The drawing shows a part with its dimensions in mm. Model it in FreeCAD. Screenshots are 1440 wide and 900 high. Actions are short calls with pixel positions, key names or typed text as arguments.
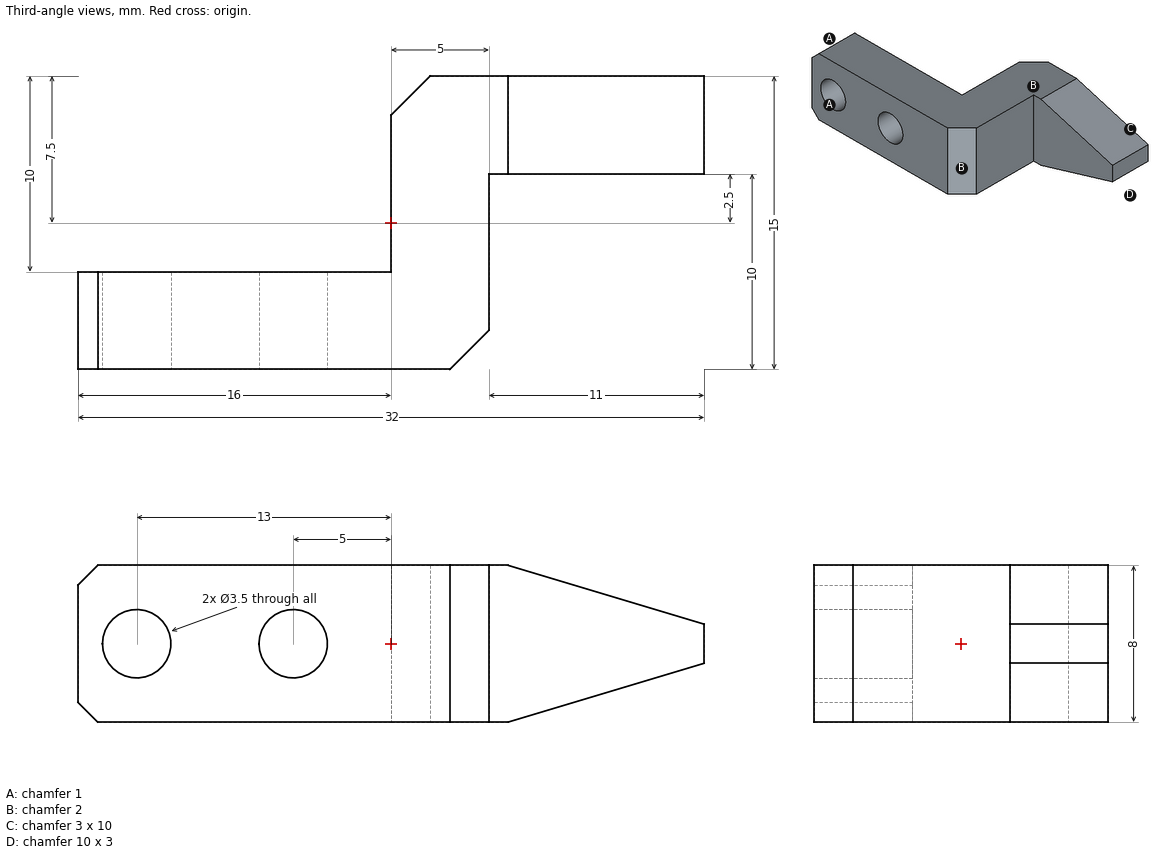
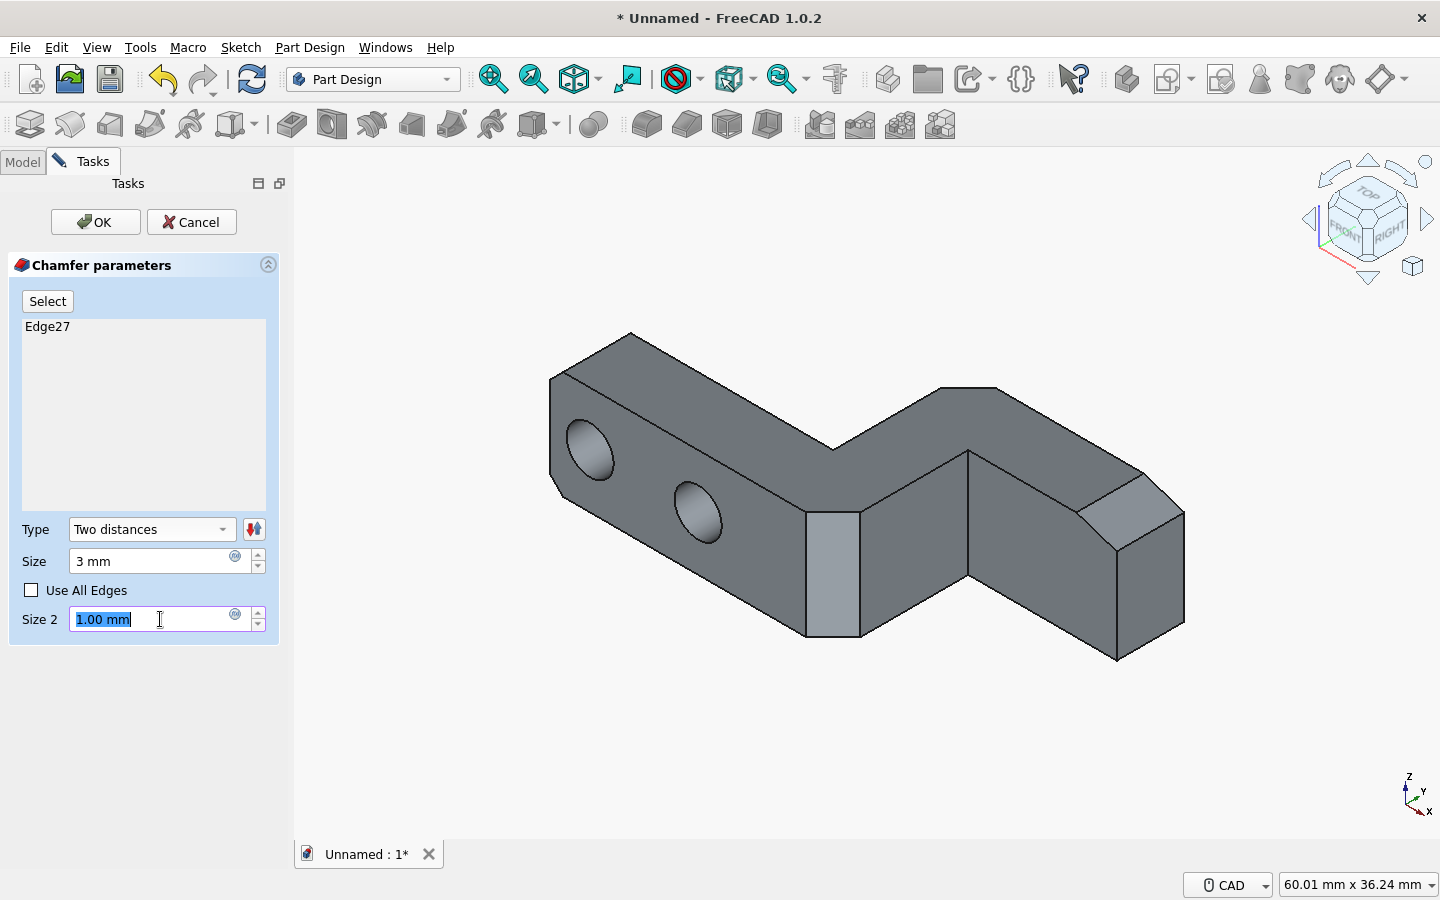
text(10)
key(Tab)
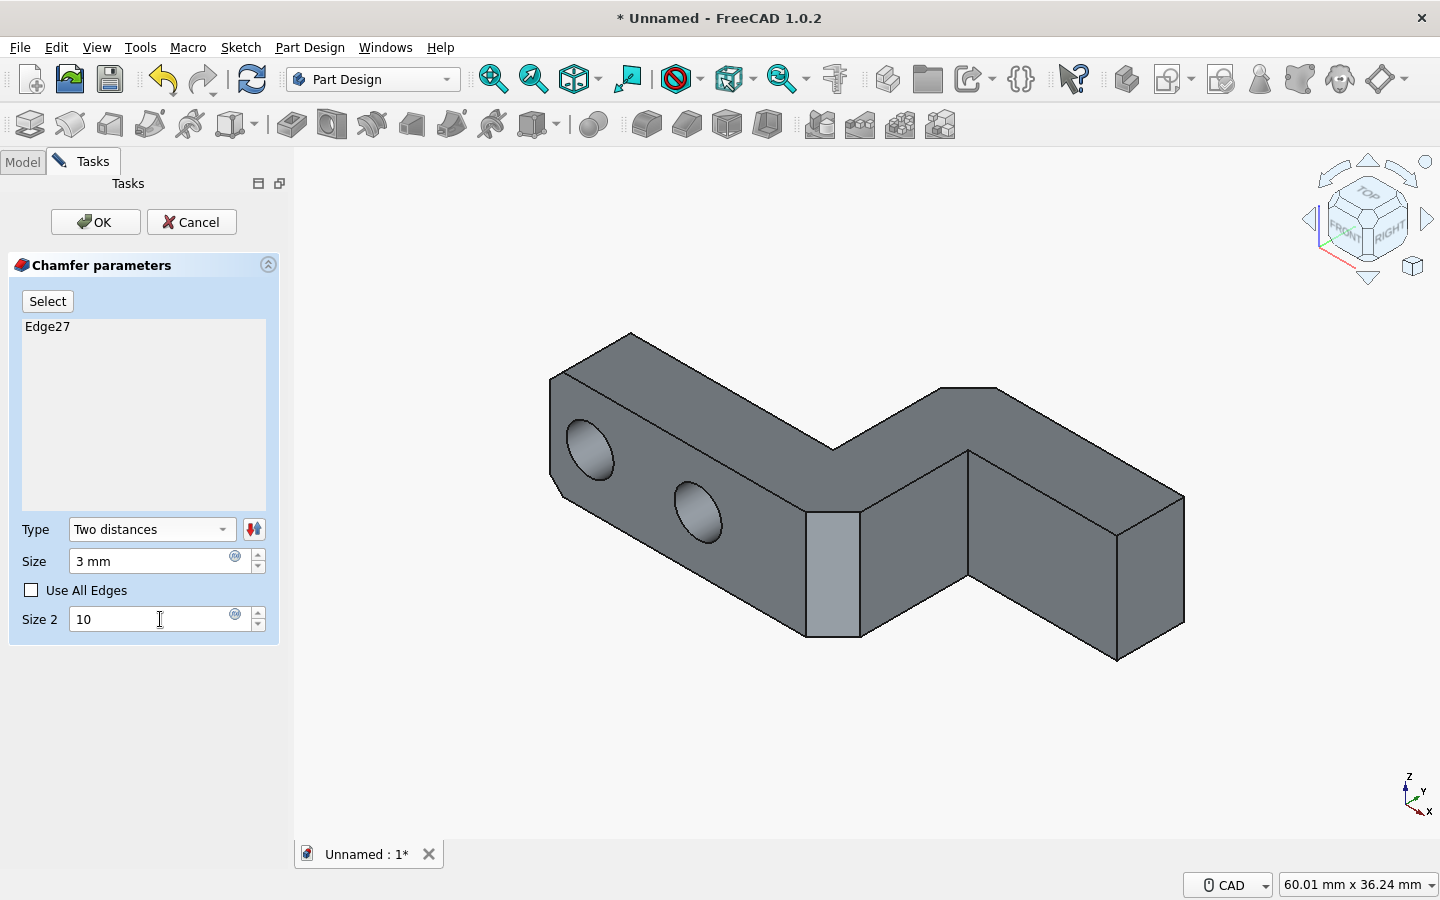
click(254, 530)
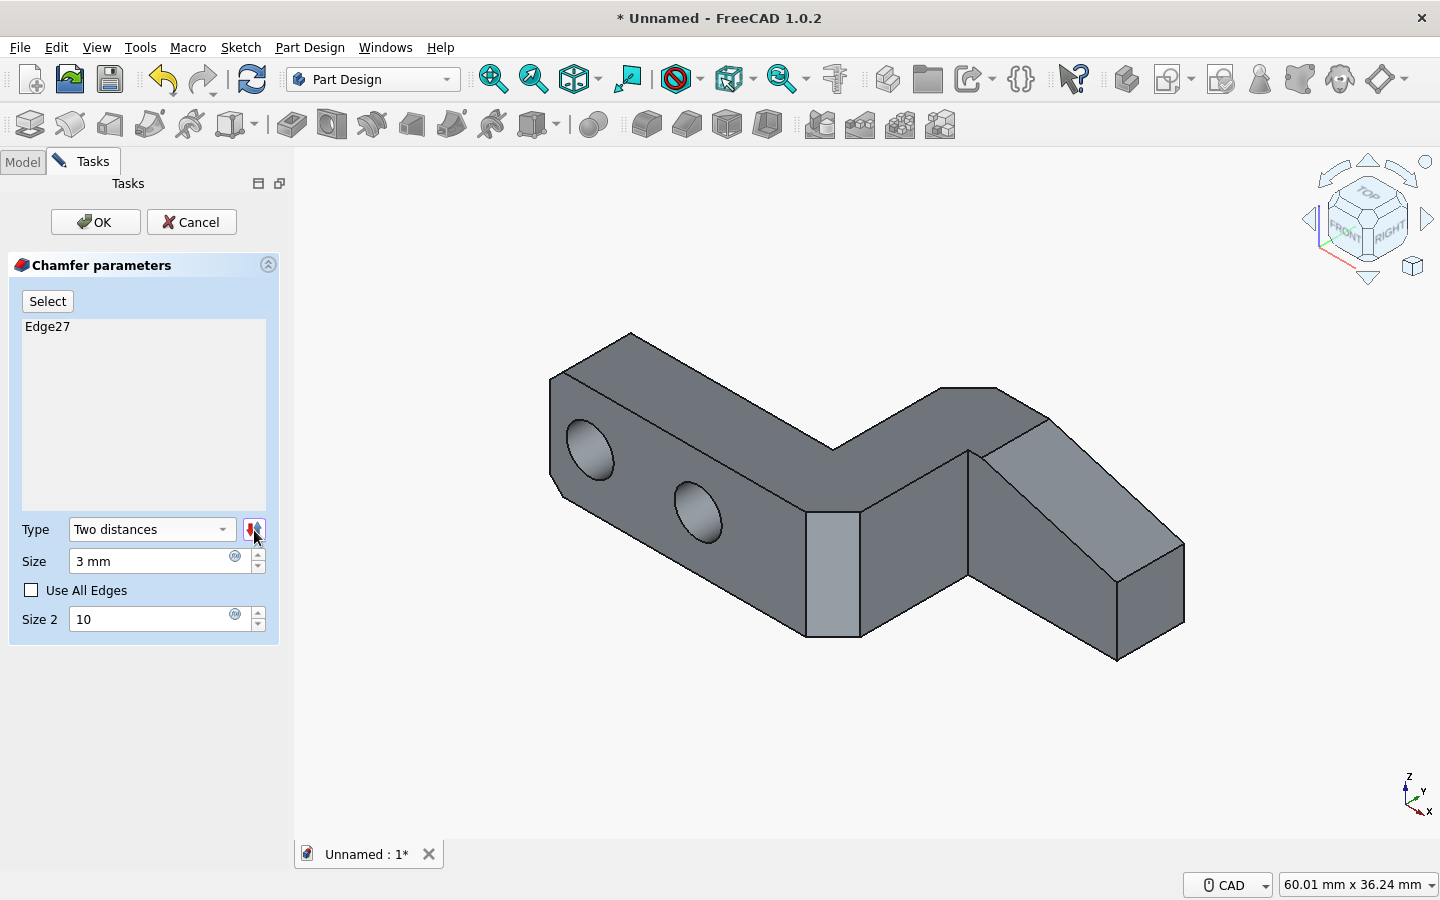
click(96, 222)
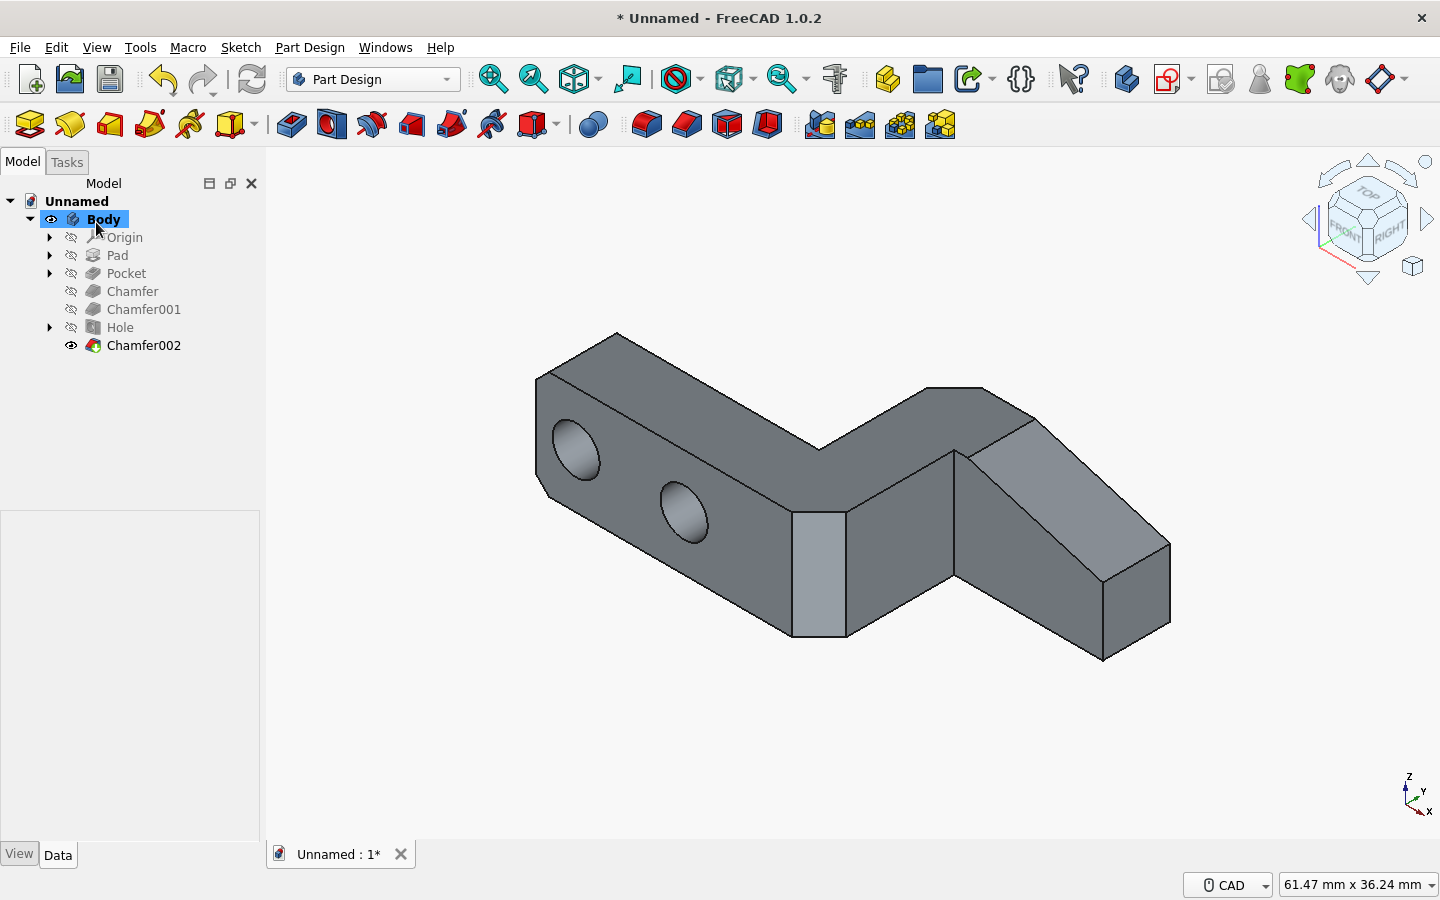
key(2)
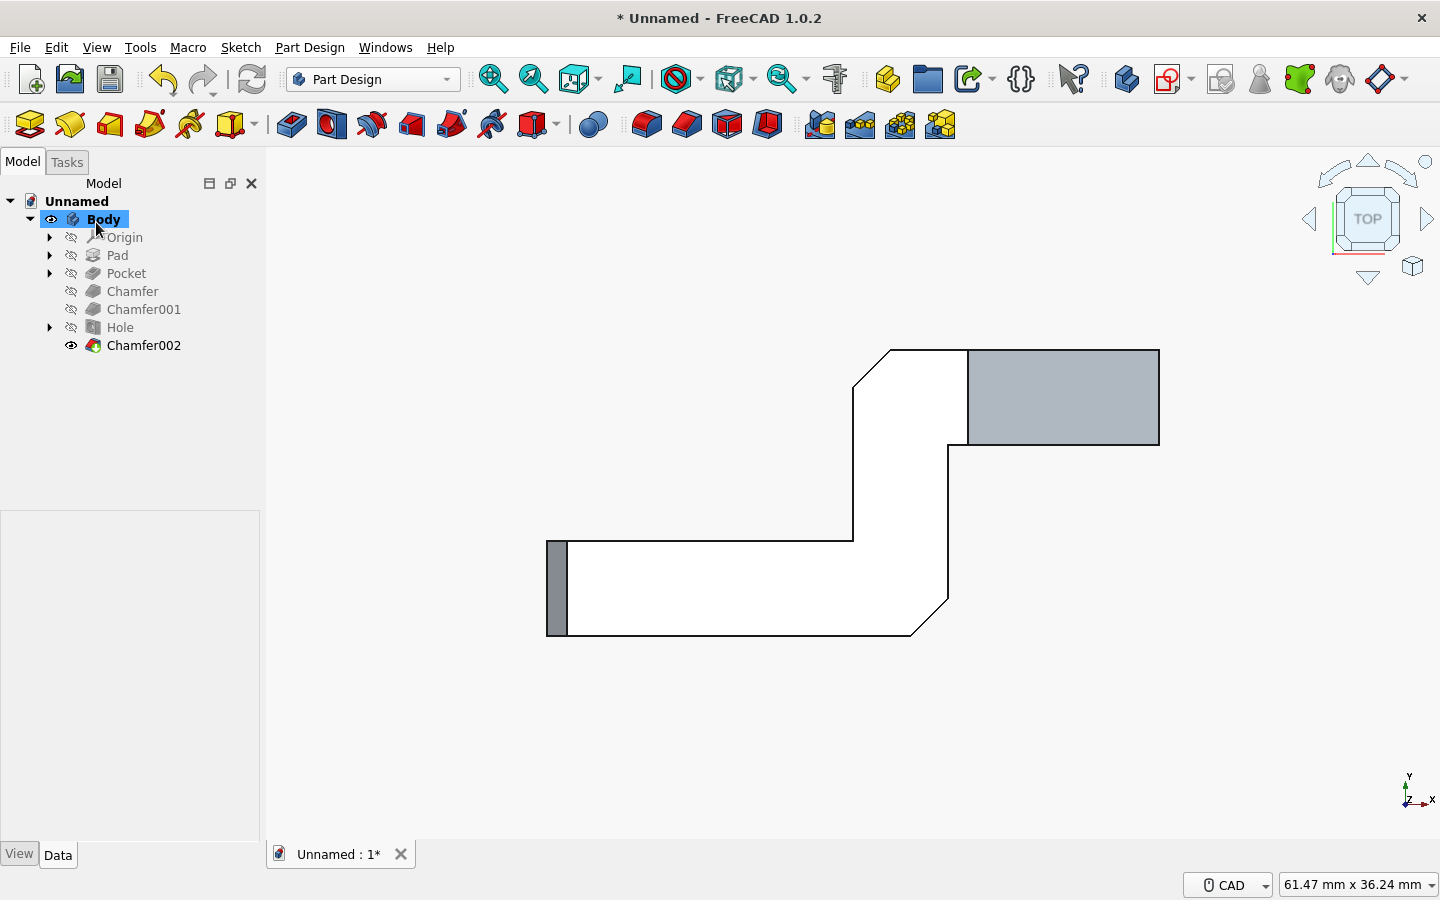
key(0)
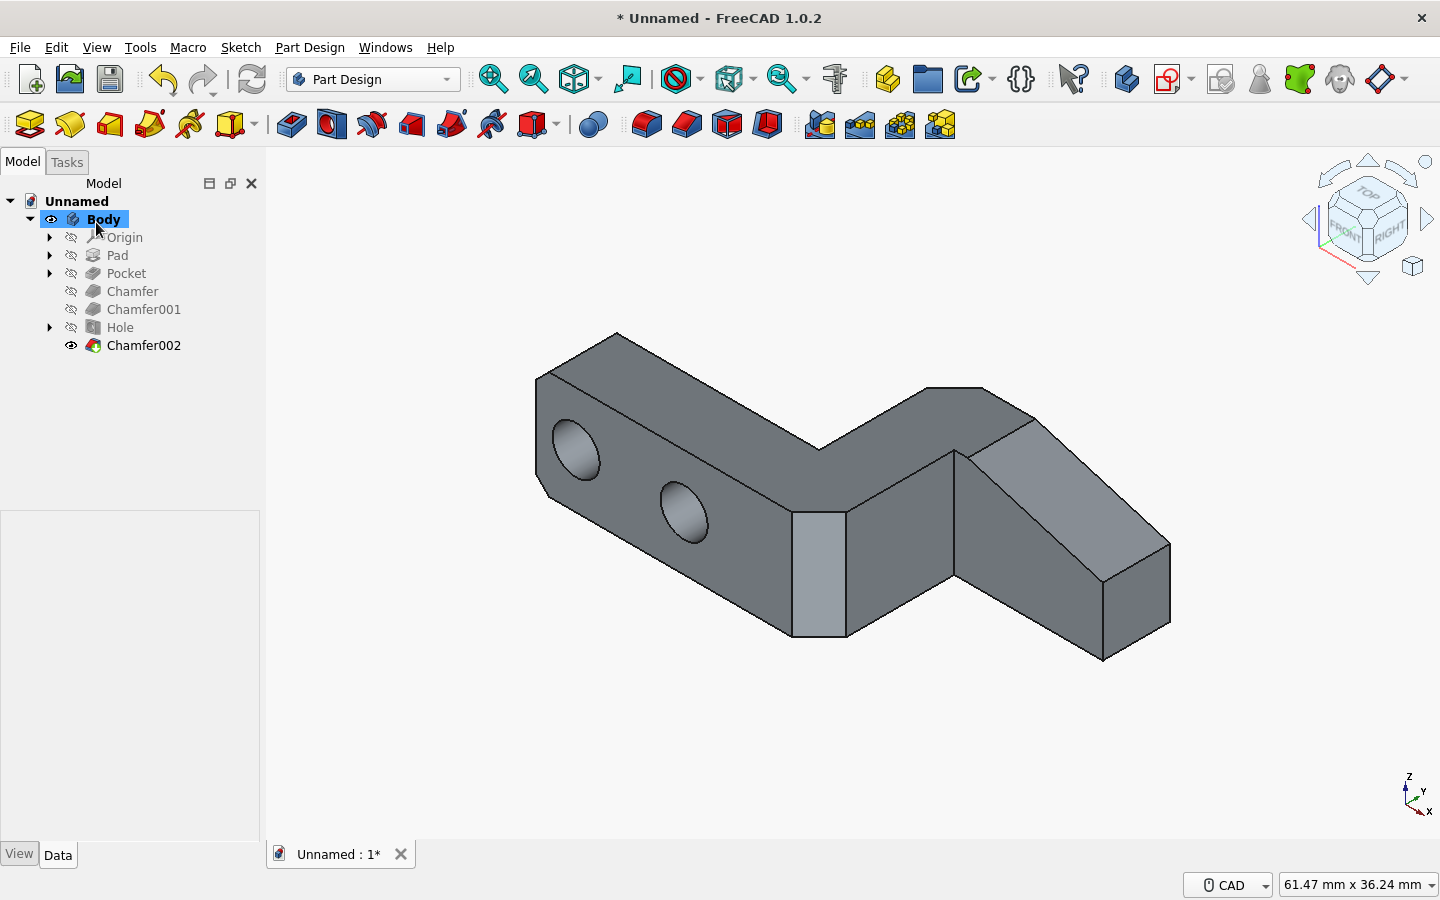
key(1)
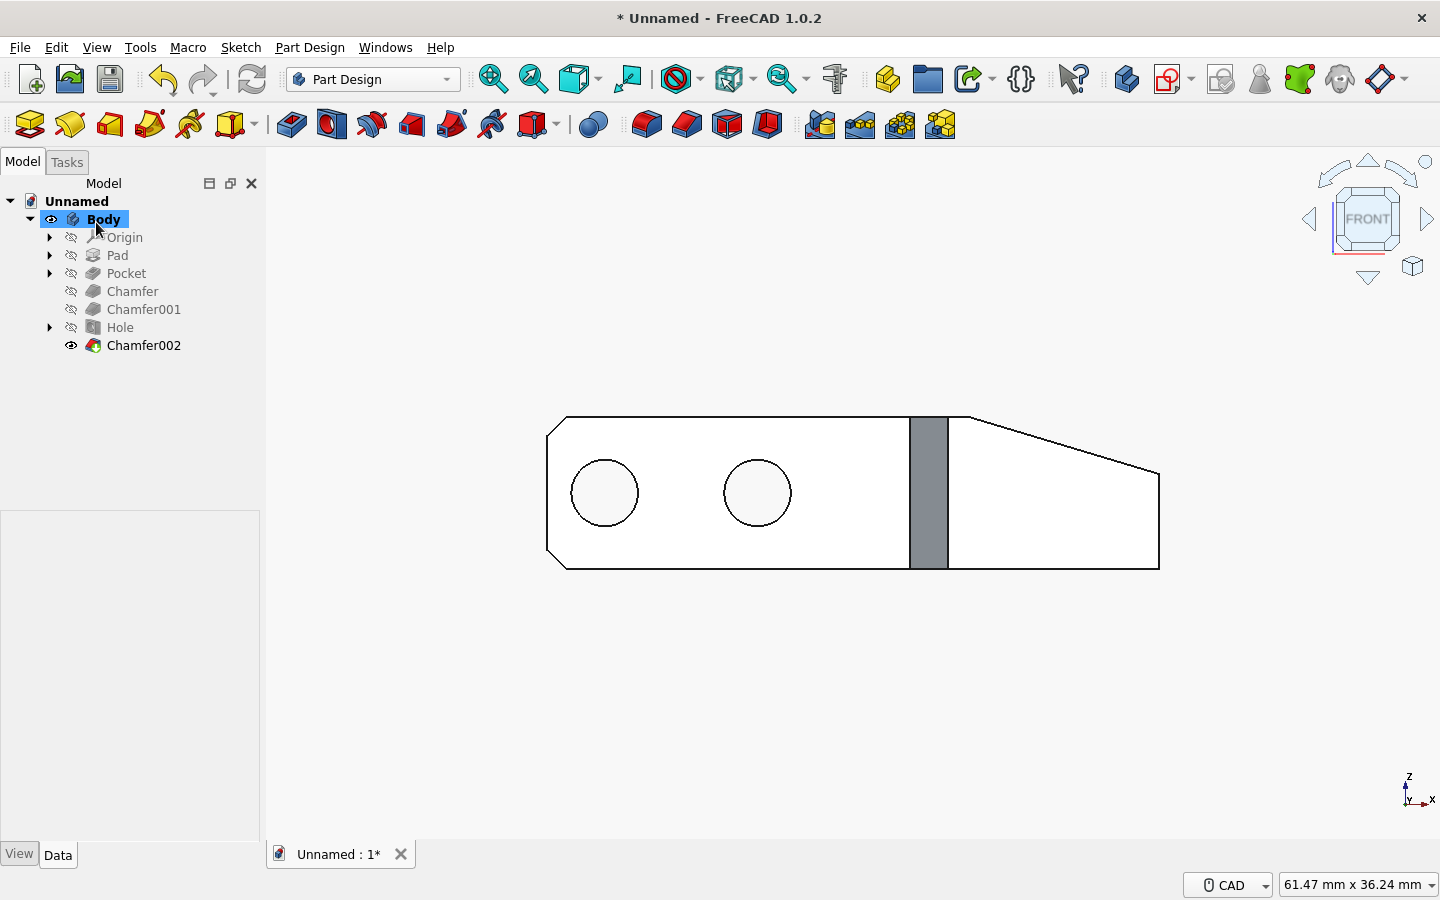
key(3)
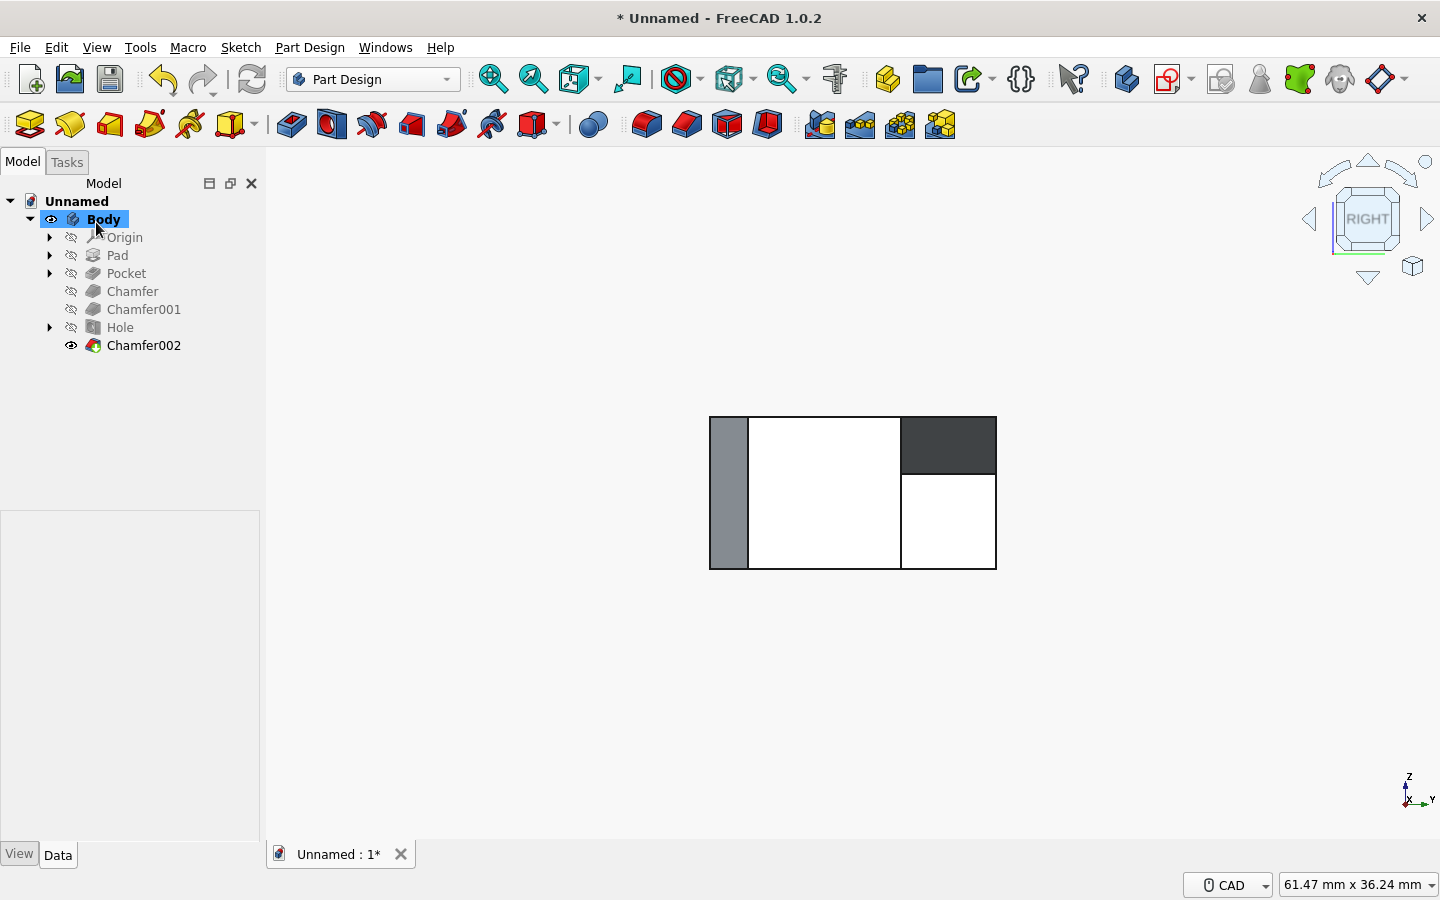
key(v)
key(f)